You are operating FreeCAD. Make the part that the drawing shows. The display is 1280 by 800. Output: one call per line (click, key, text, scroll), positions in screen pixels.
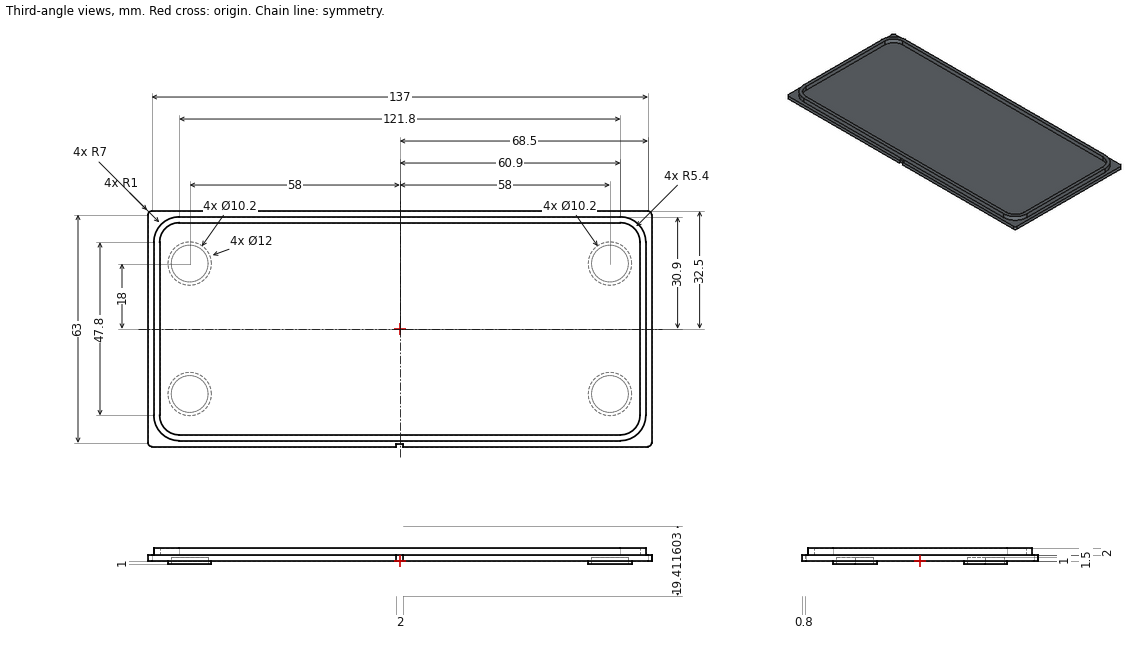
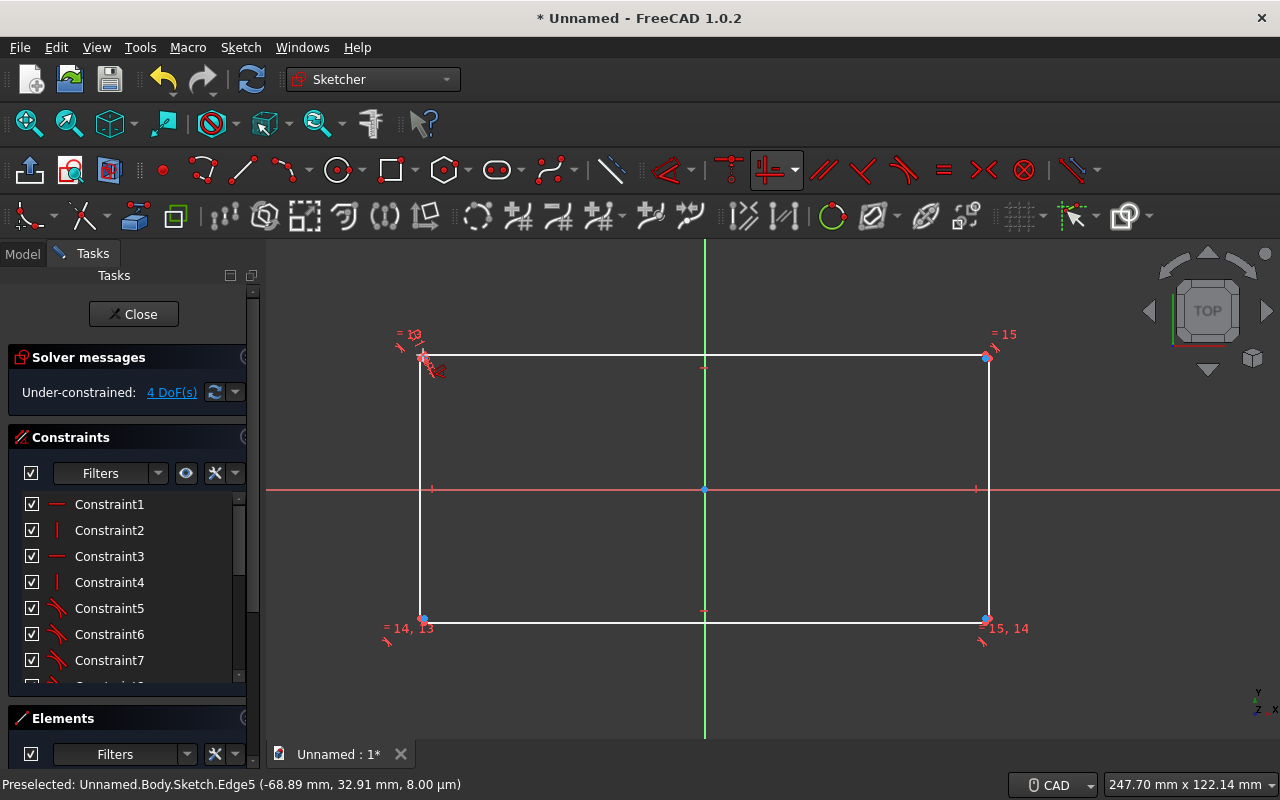
click(420, 437)
click(386, 429)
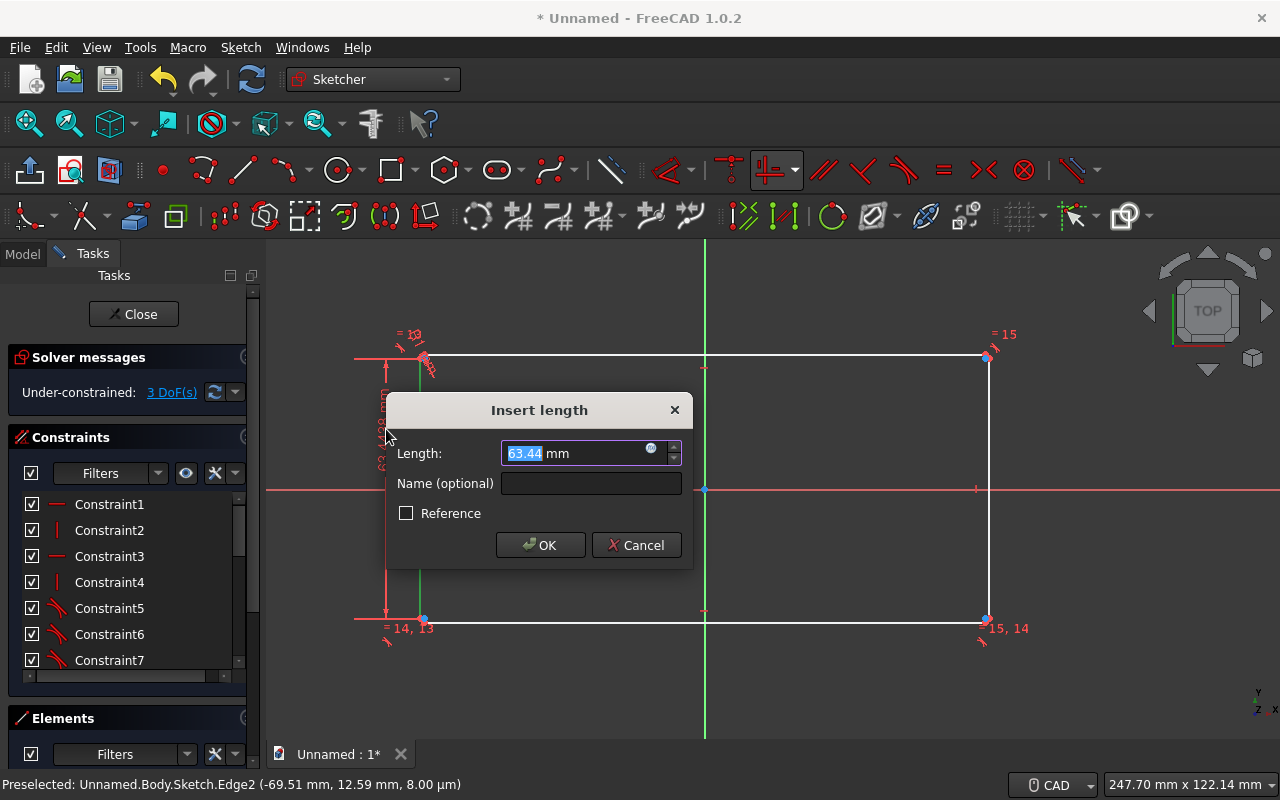
text(63)
key(Return)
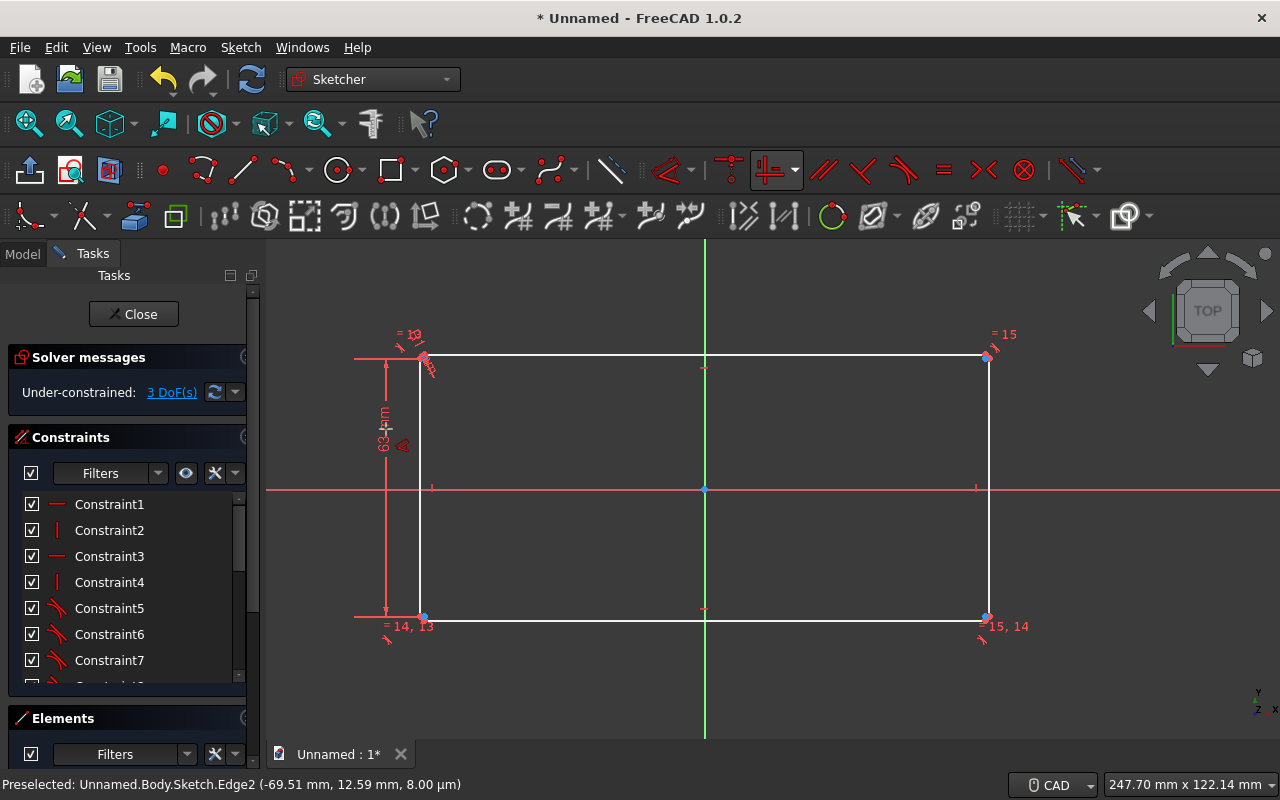
click(817, 355)
click(576, 321)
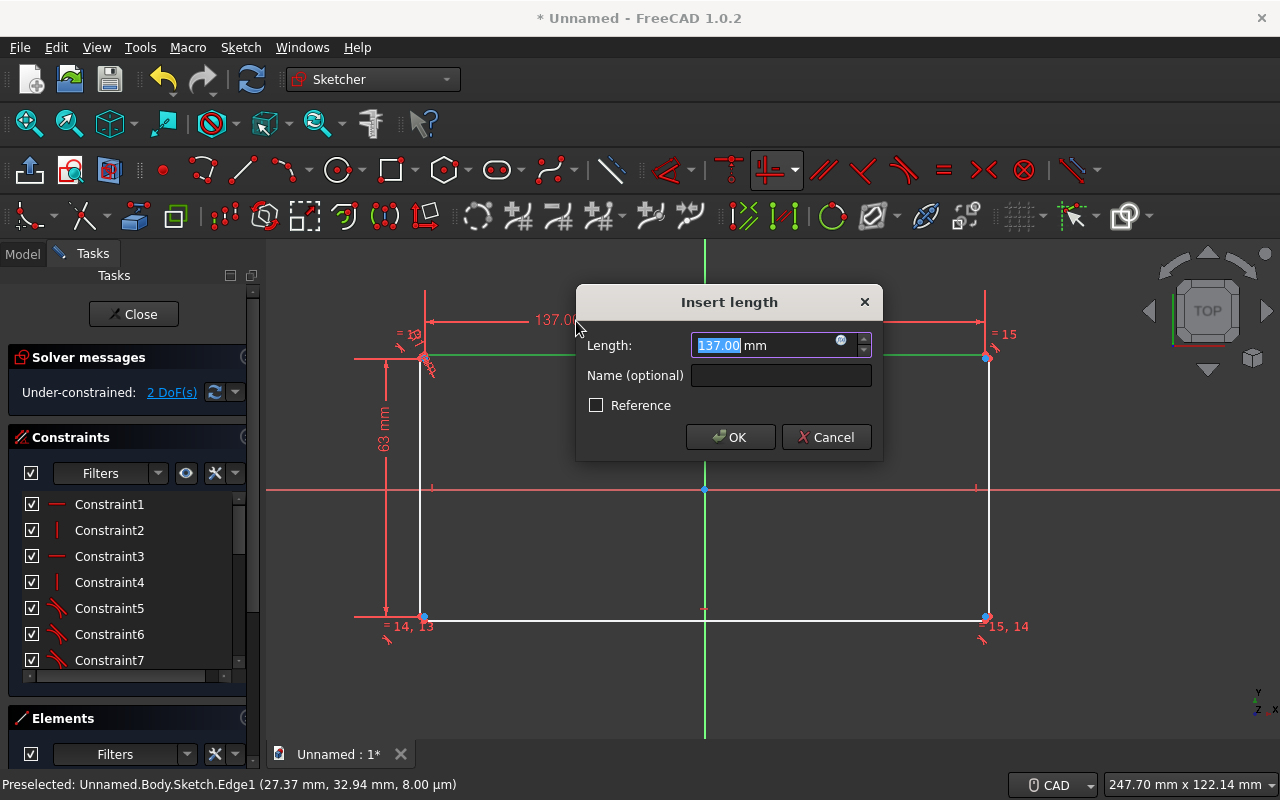
text(137)
key(Return)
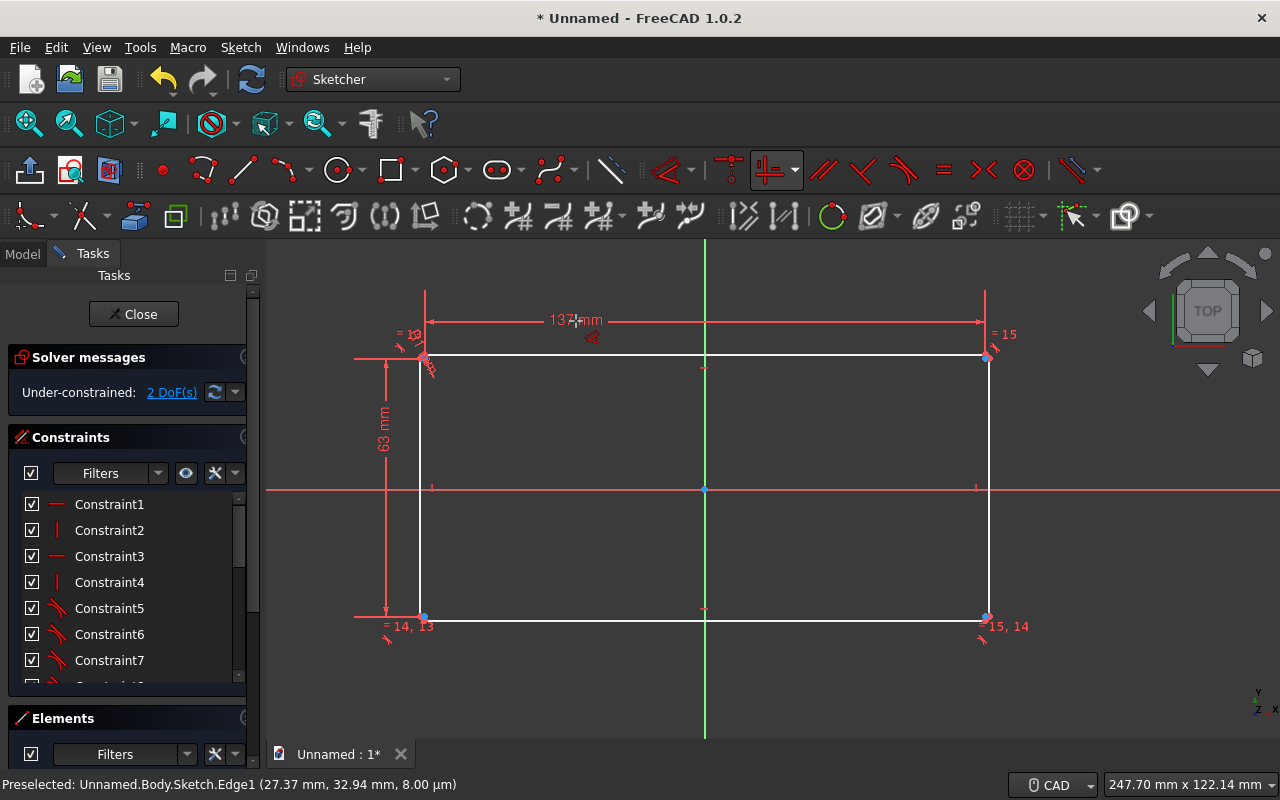
scroll(985, 355, up, 6)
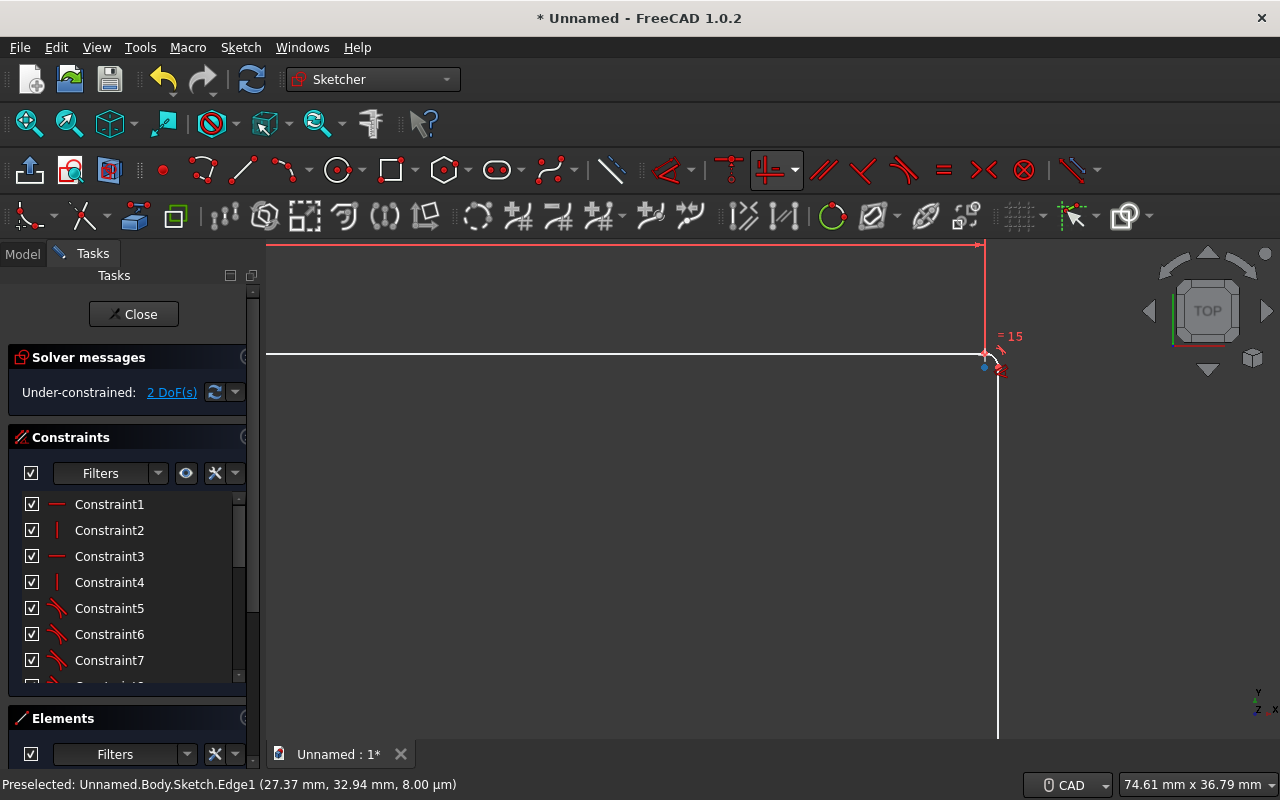
click(985, 353)
click(639, 319)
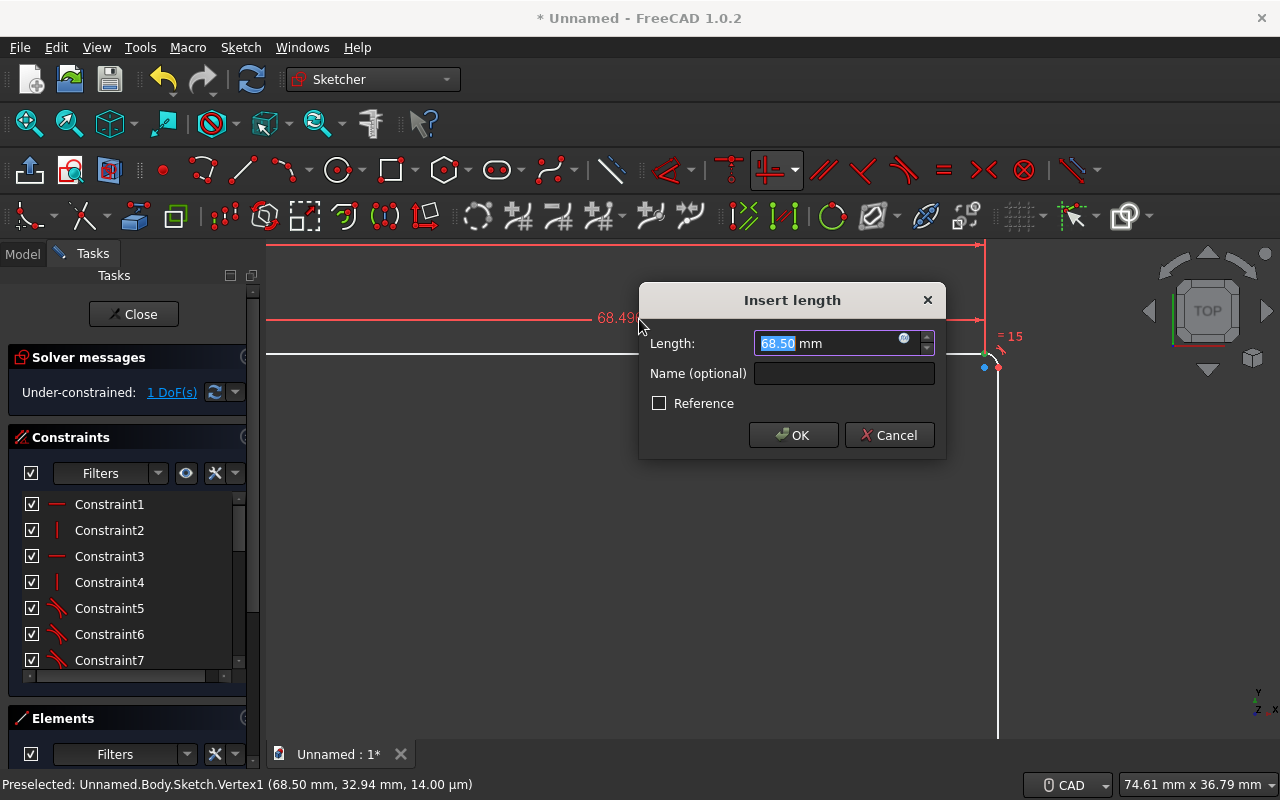
text(68.5)
key(Return)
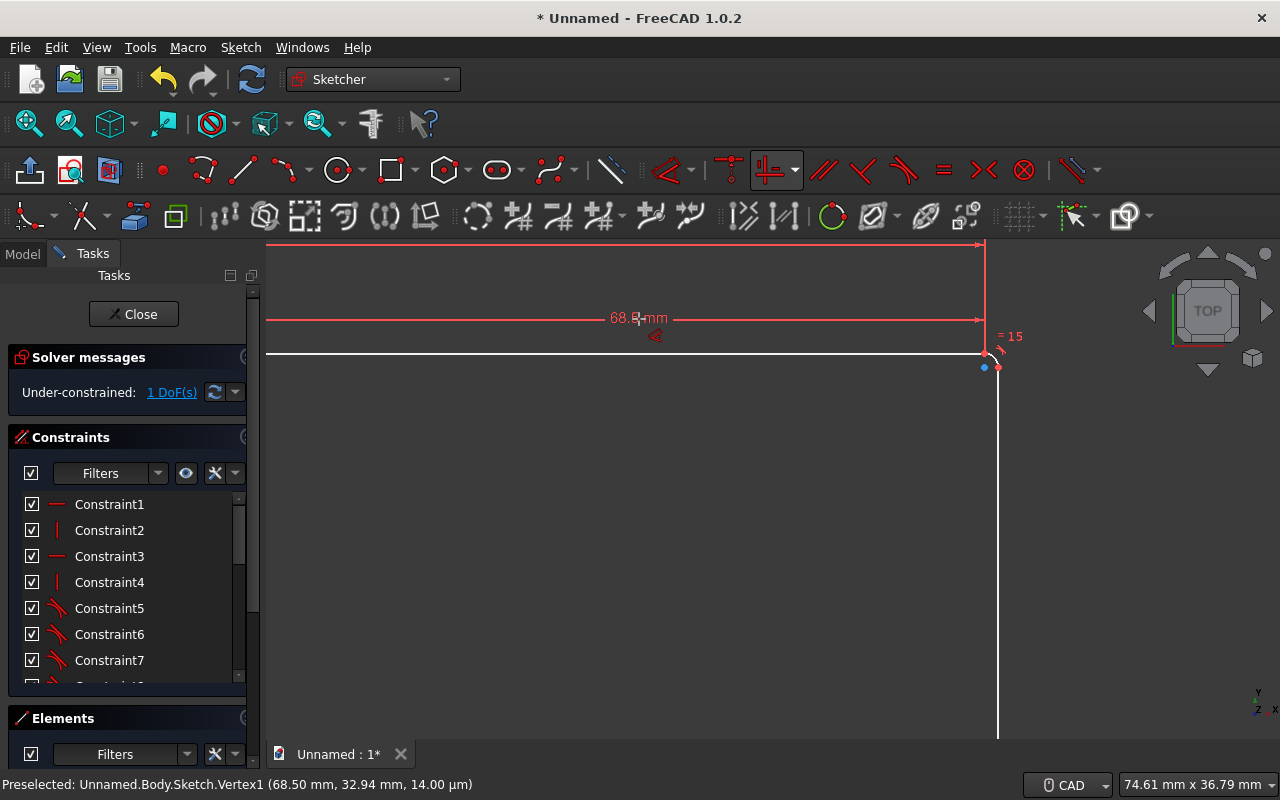
click(985, 353)
click(1019, 532)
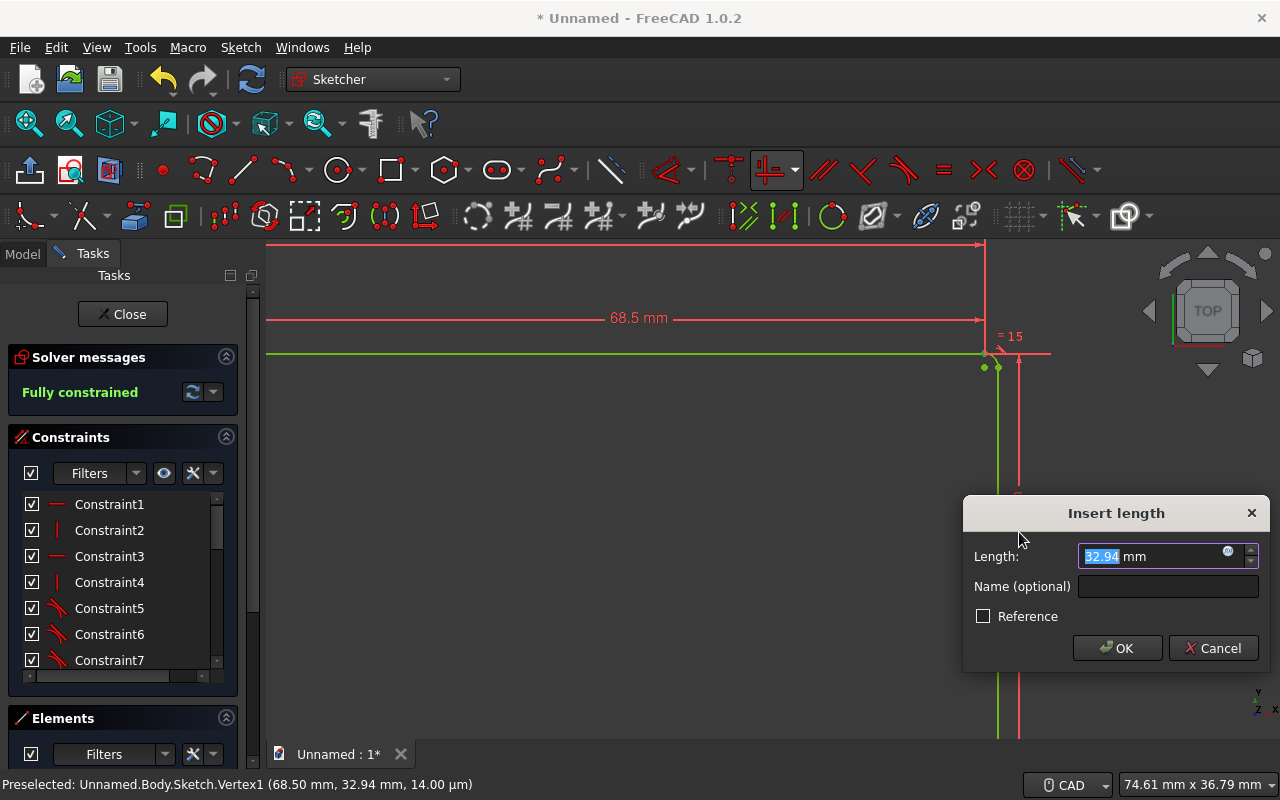
text(32.5)
key(Return)
key(Escape)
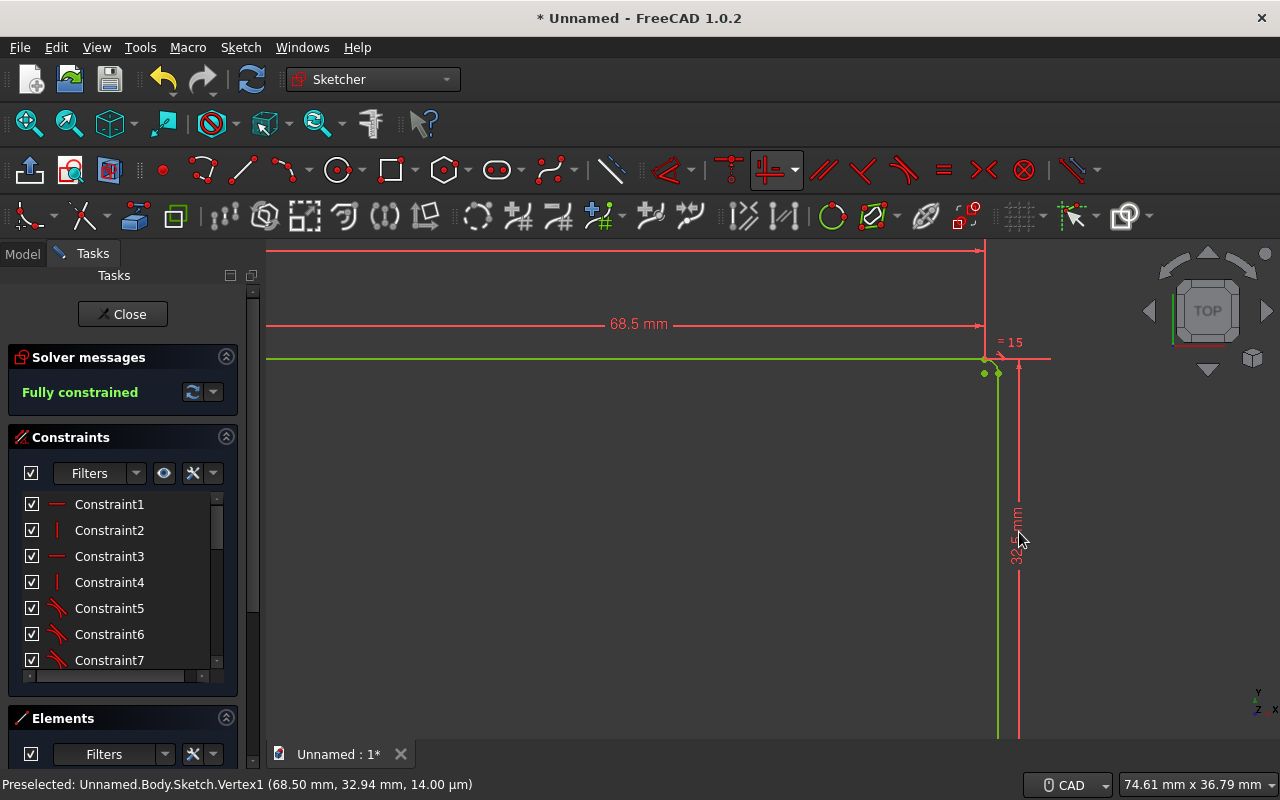
click(123, 314)